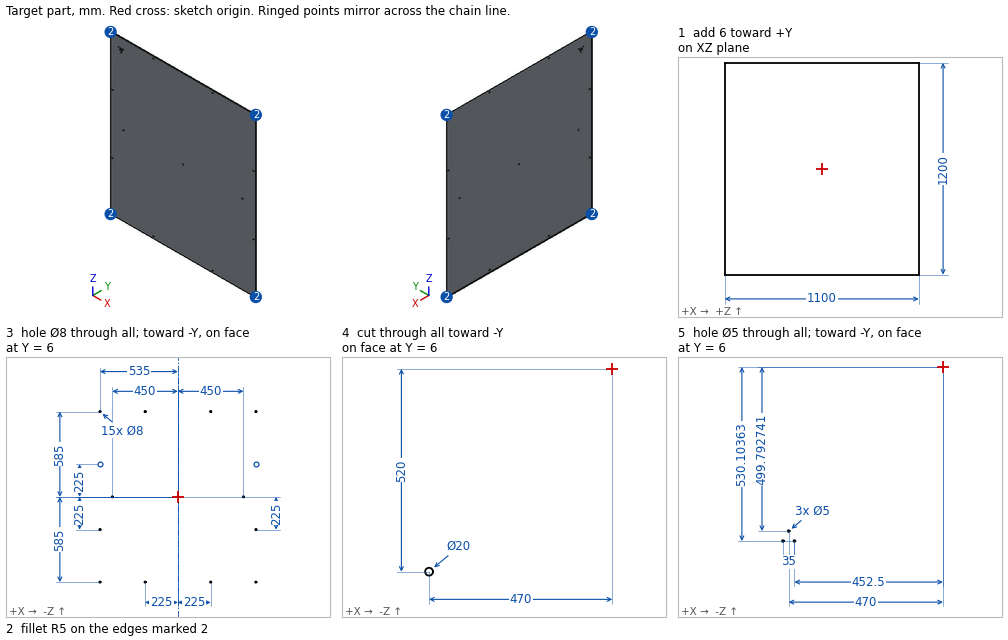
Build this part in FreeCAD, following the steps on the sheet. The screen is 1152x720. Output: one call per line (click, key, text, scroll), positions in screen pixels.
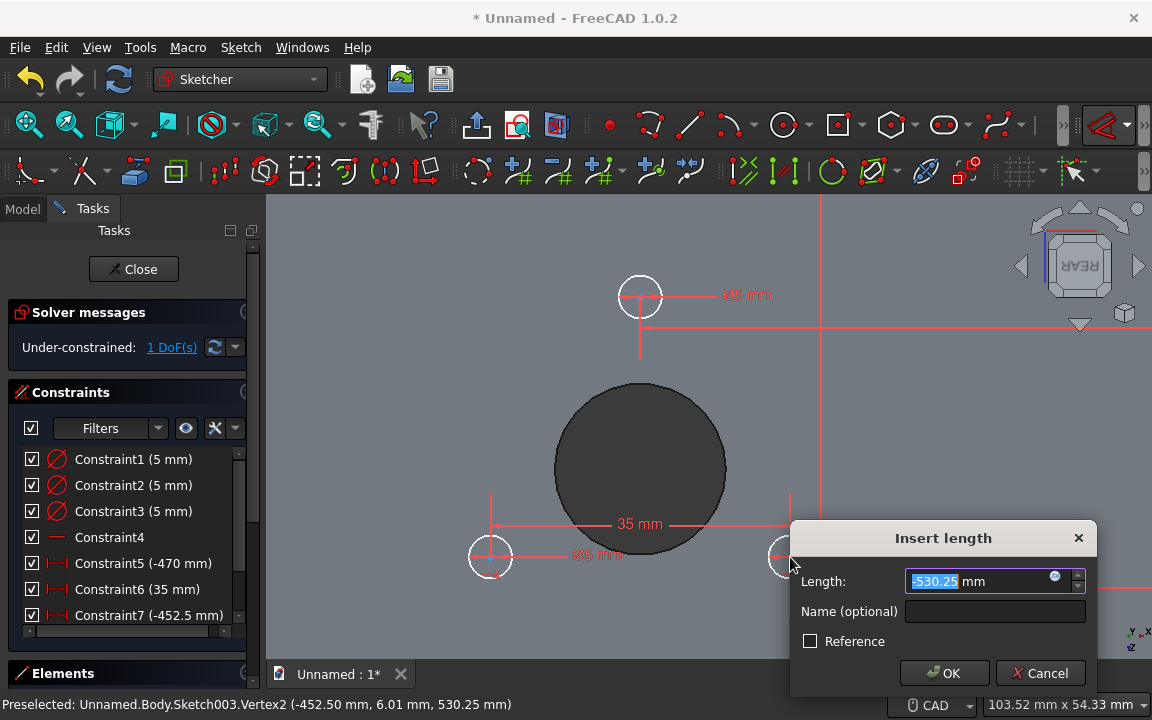
text(-530.10363)
key(Return)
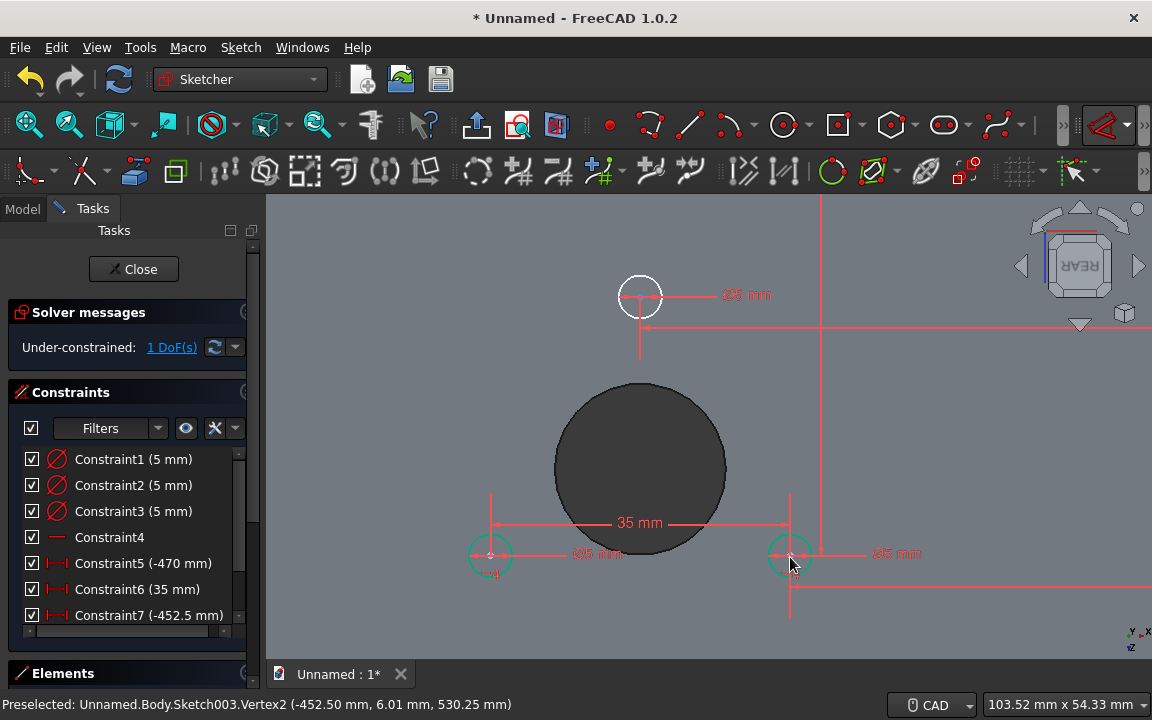
click(640, 297)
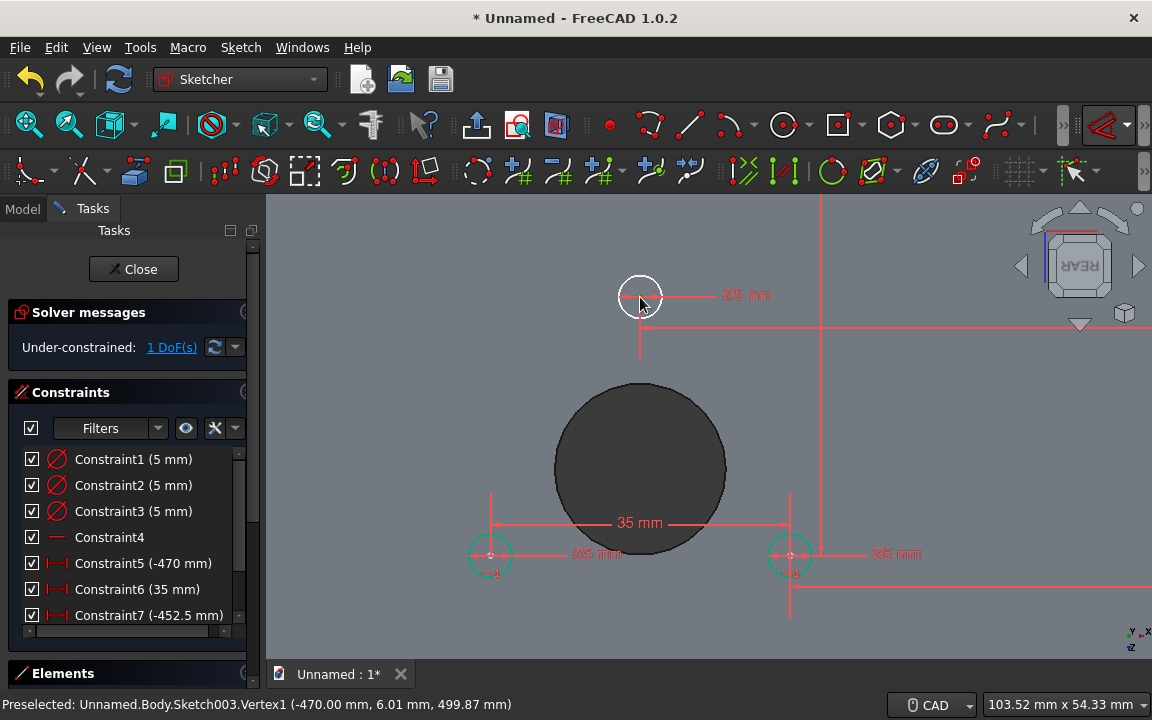
click(1130, 126)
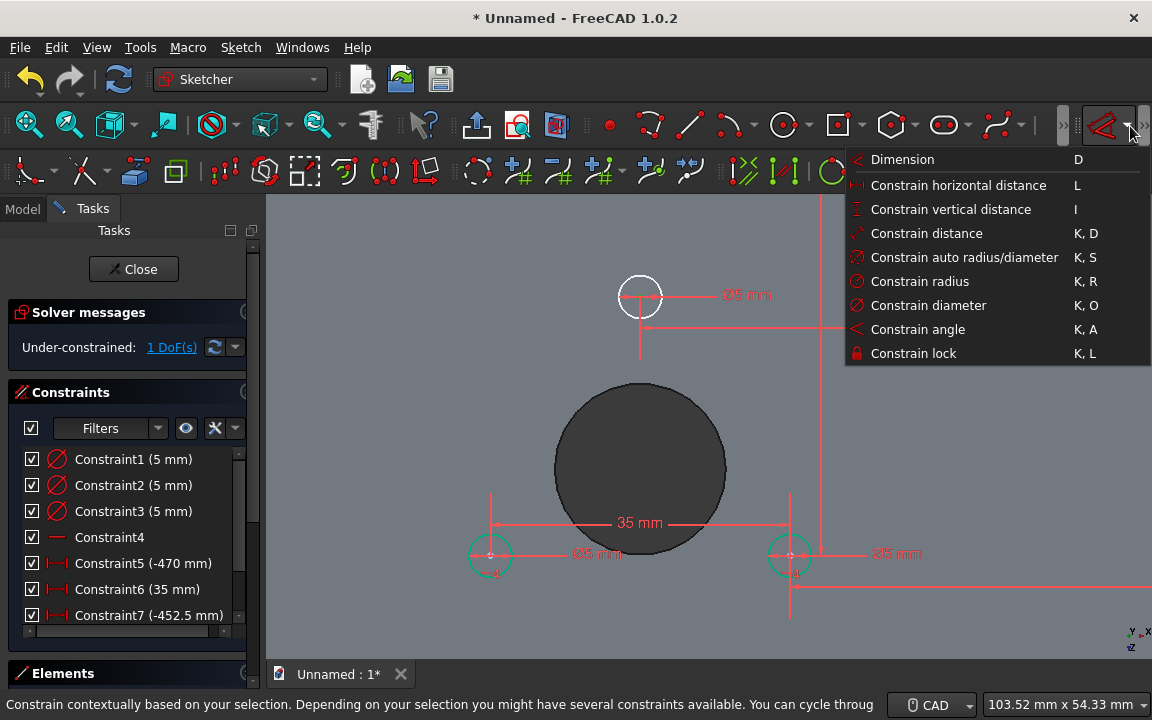
click(998, 209)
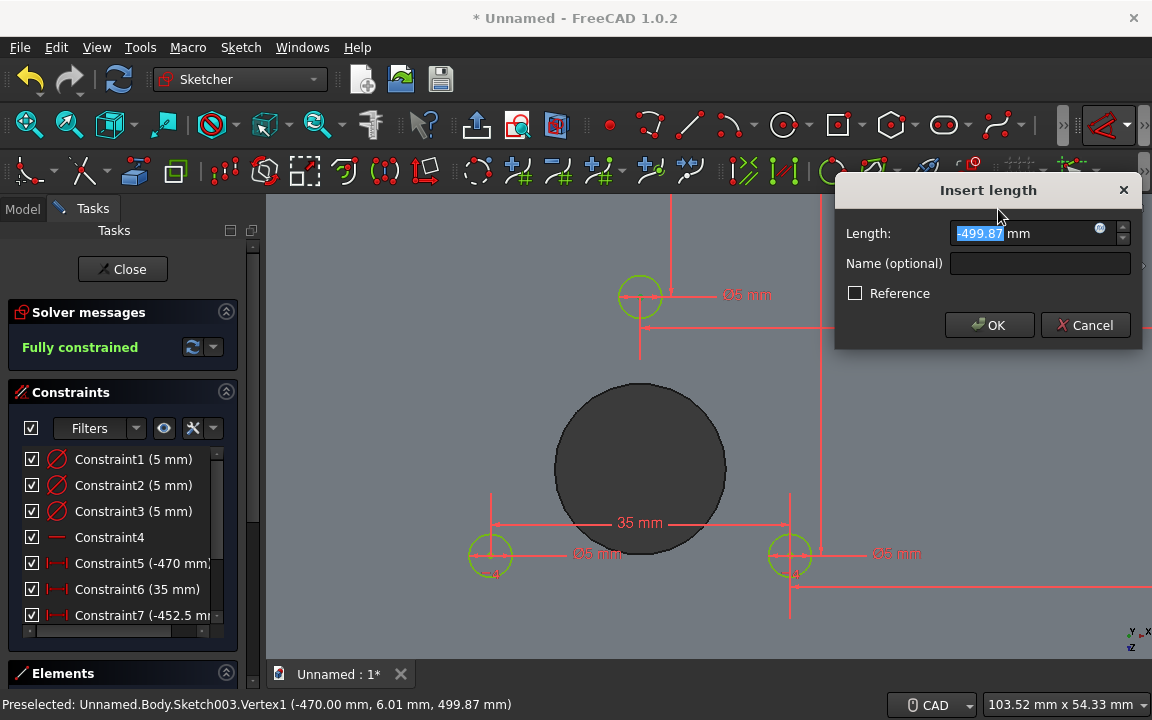
text(-499.792741)
key(Return)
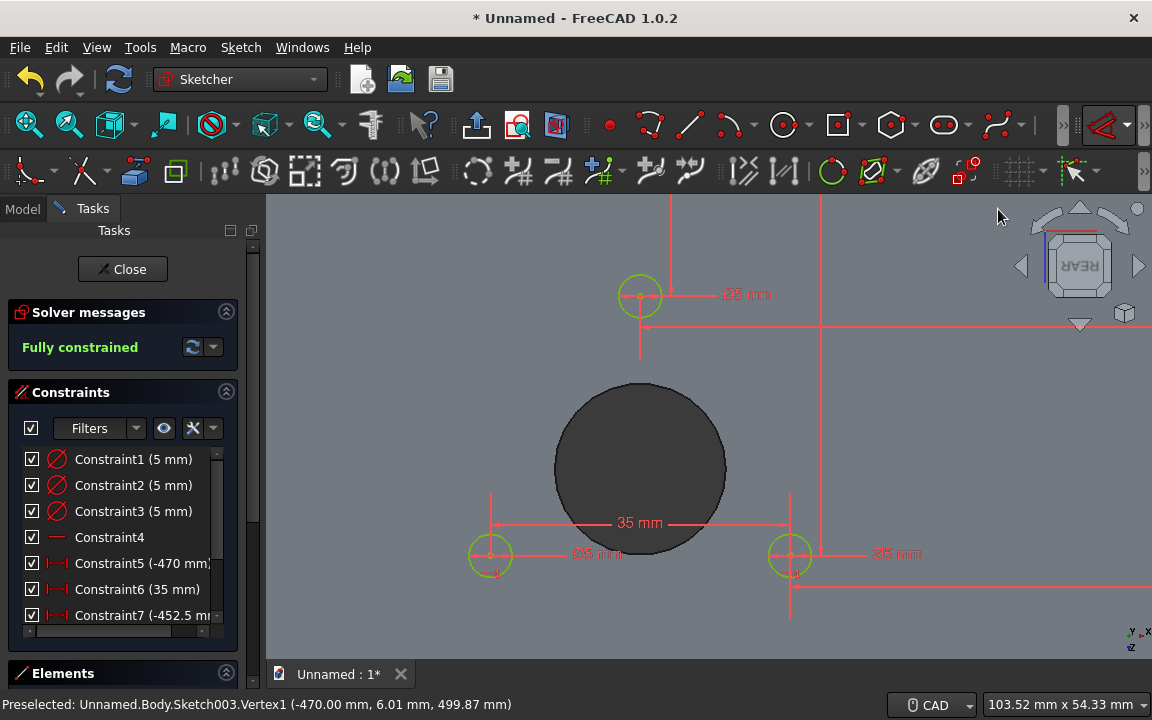
click(123, 269)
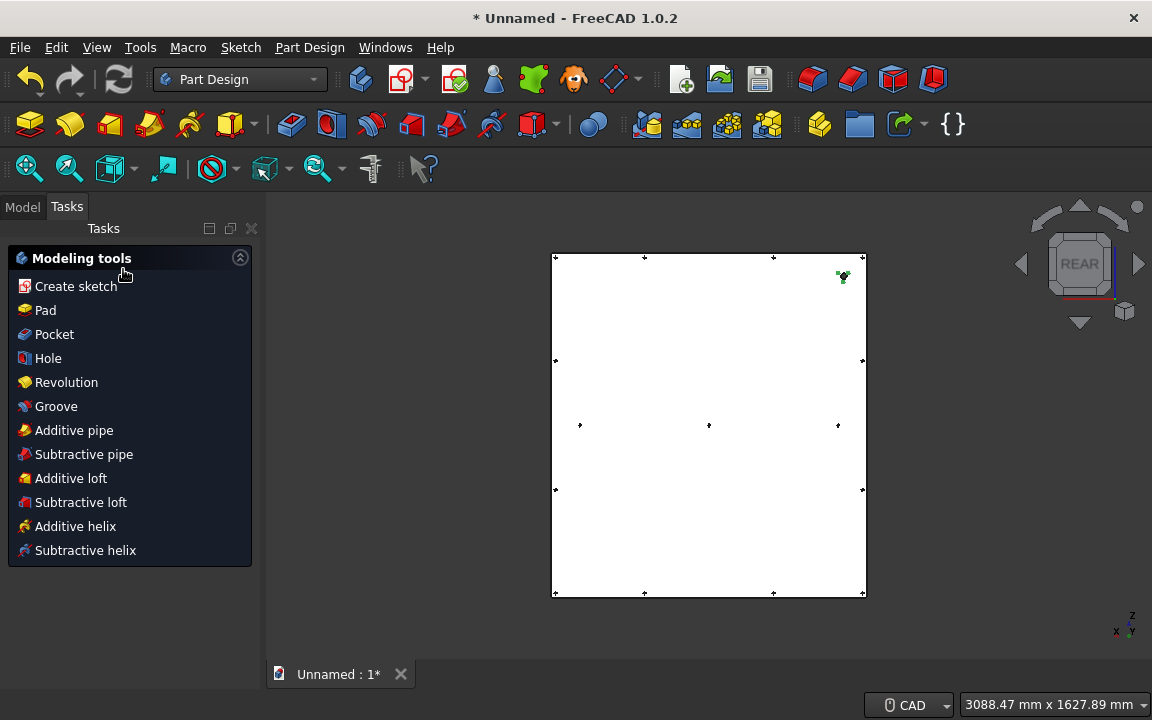
click(332, 124)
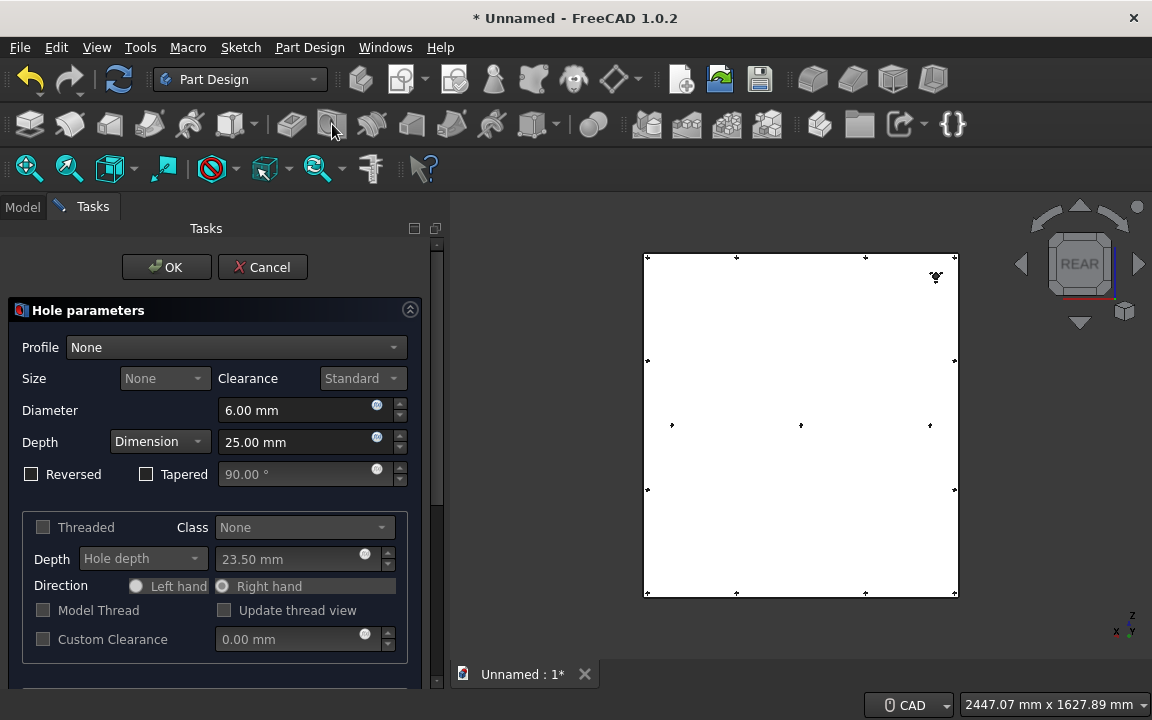
triple_click(305, 410)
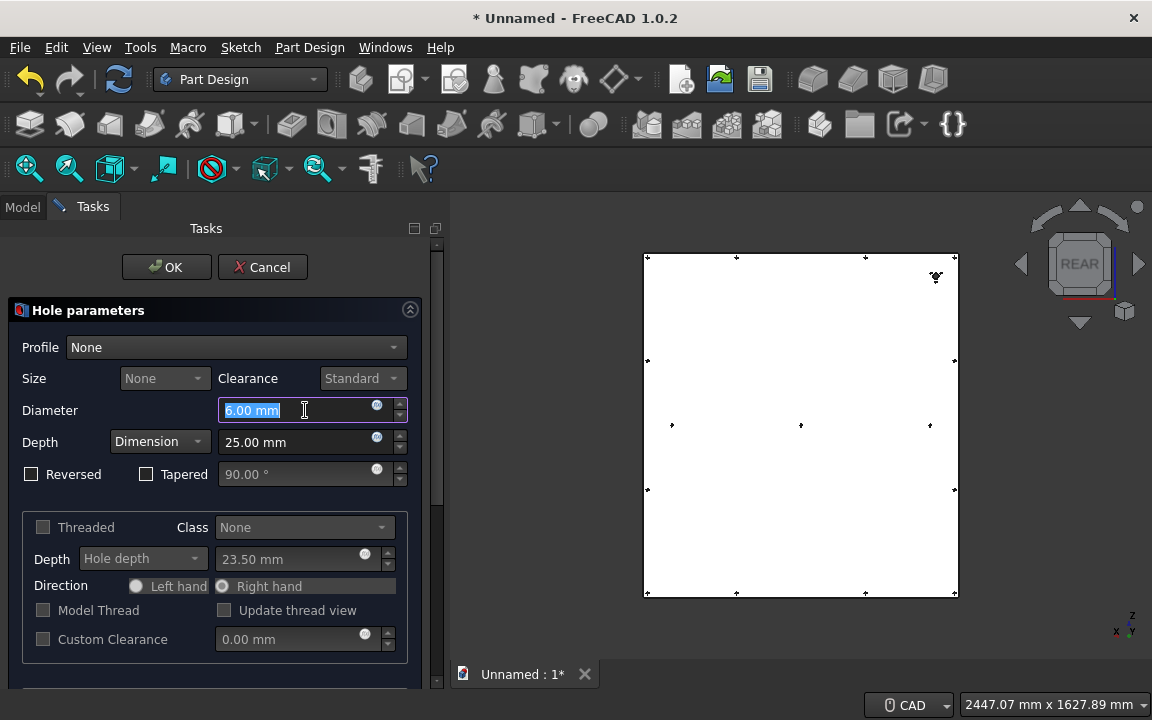
text(5)
key(Tab)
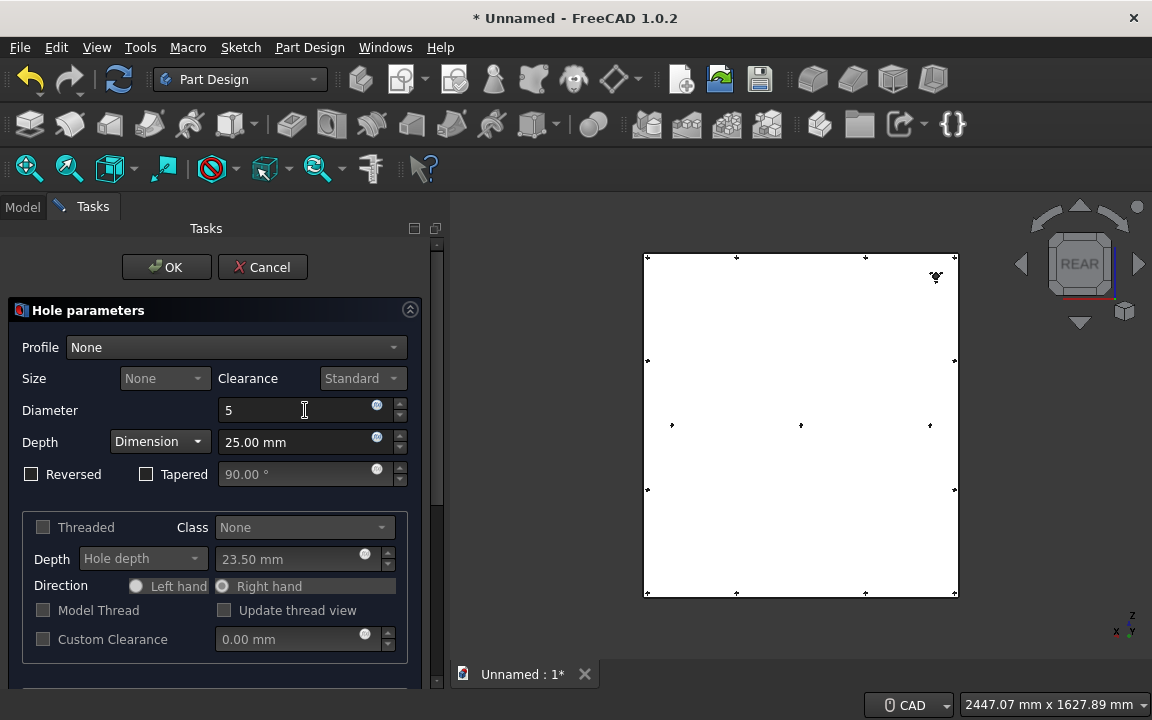
click(161, 442)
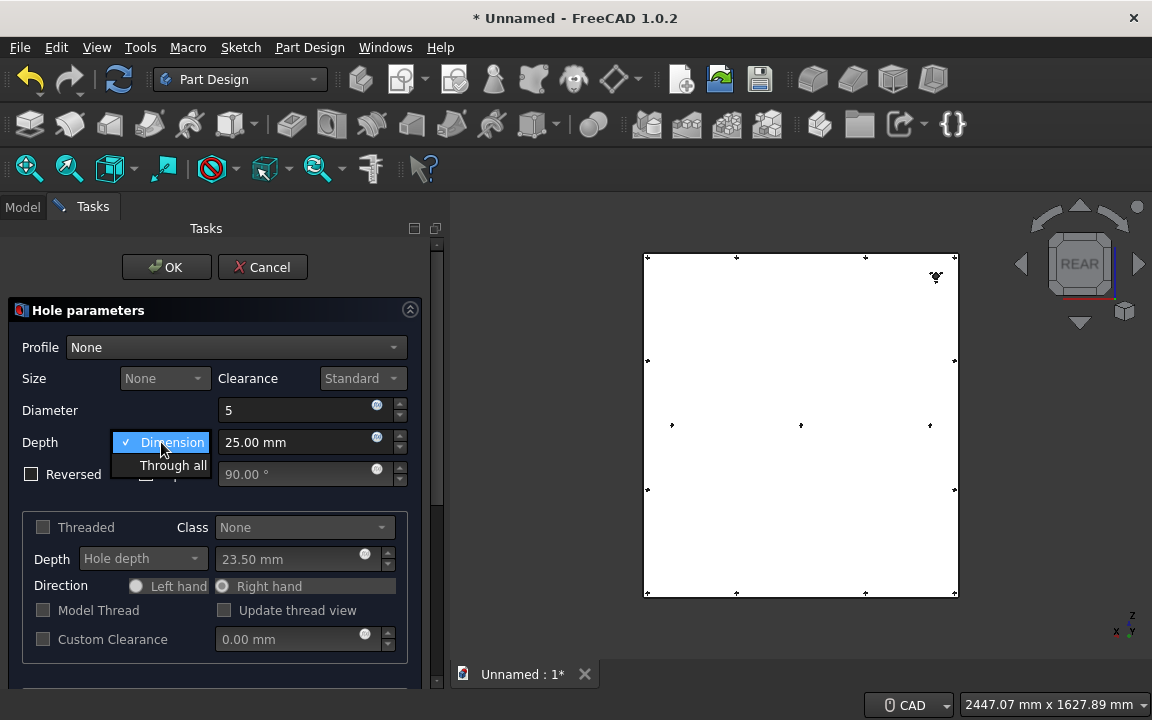
click(160, 466)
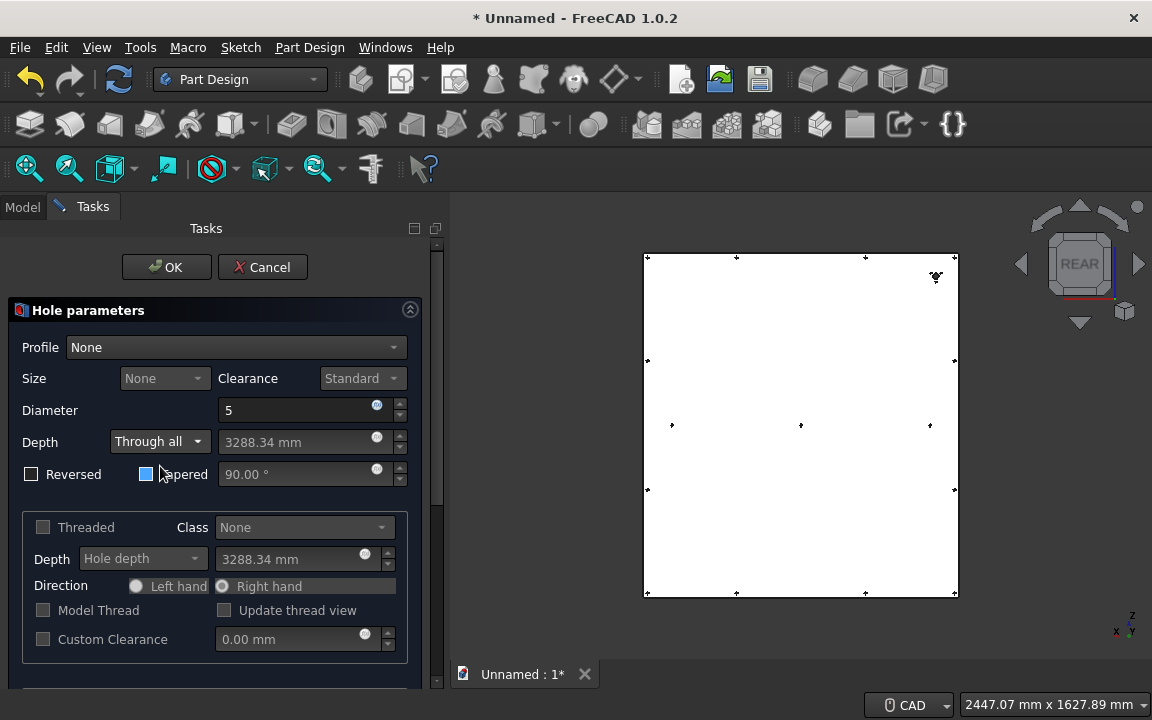
click(167, 267)